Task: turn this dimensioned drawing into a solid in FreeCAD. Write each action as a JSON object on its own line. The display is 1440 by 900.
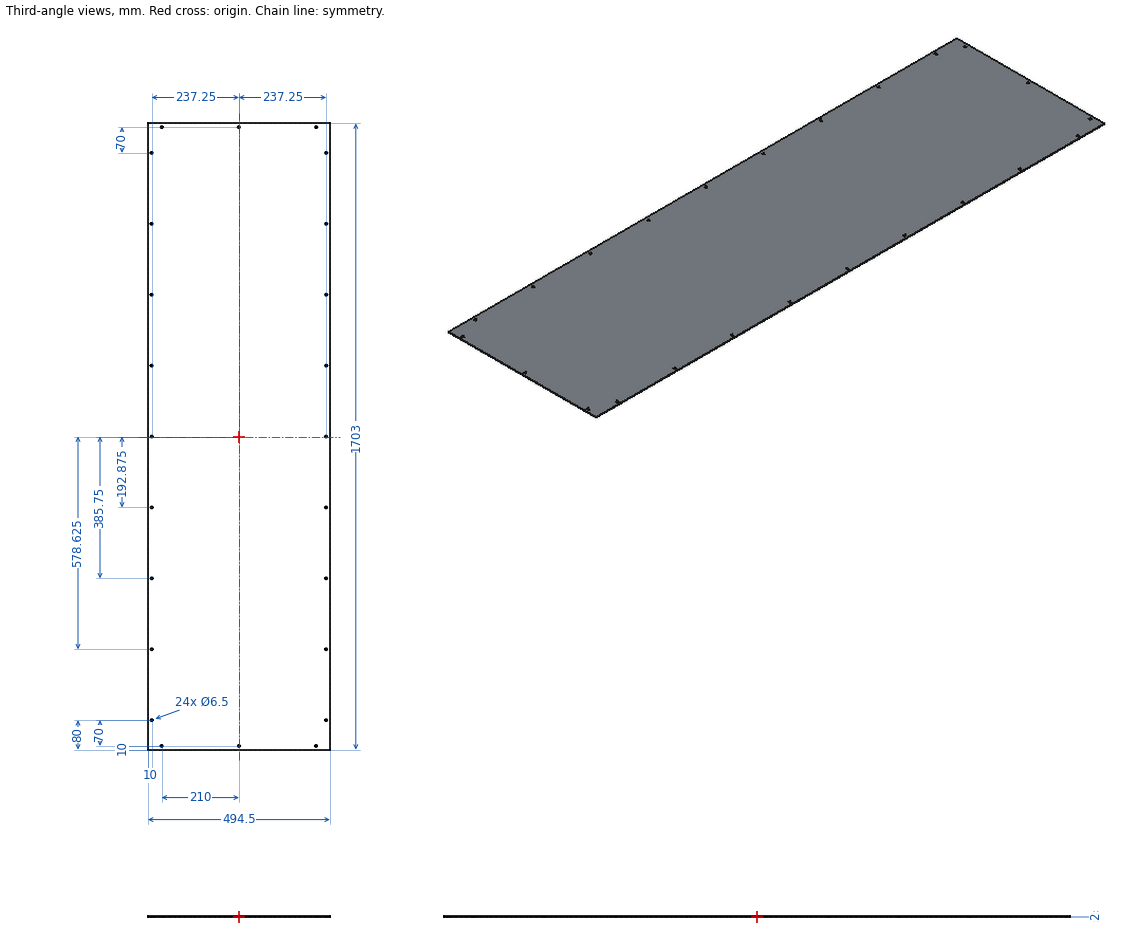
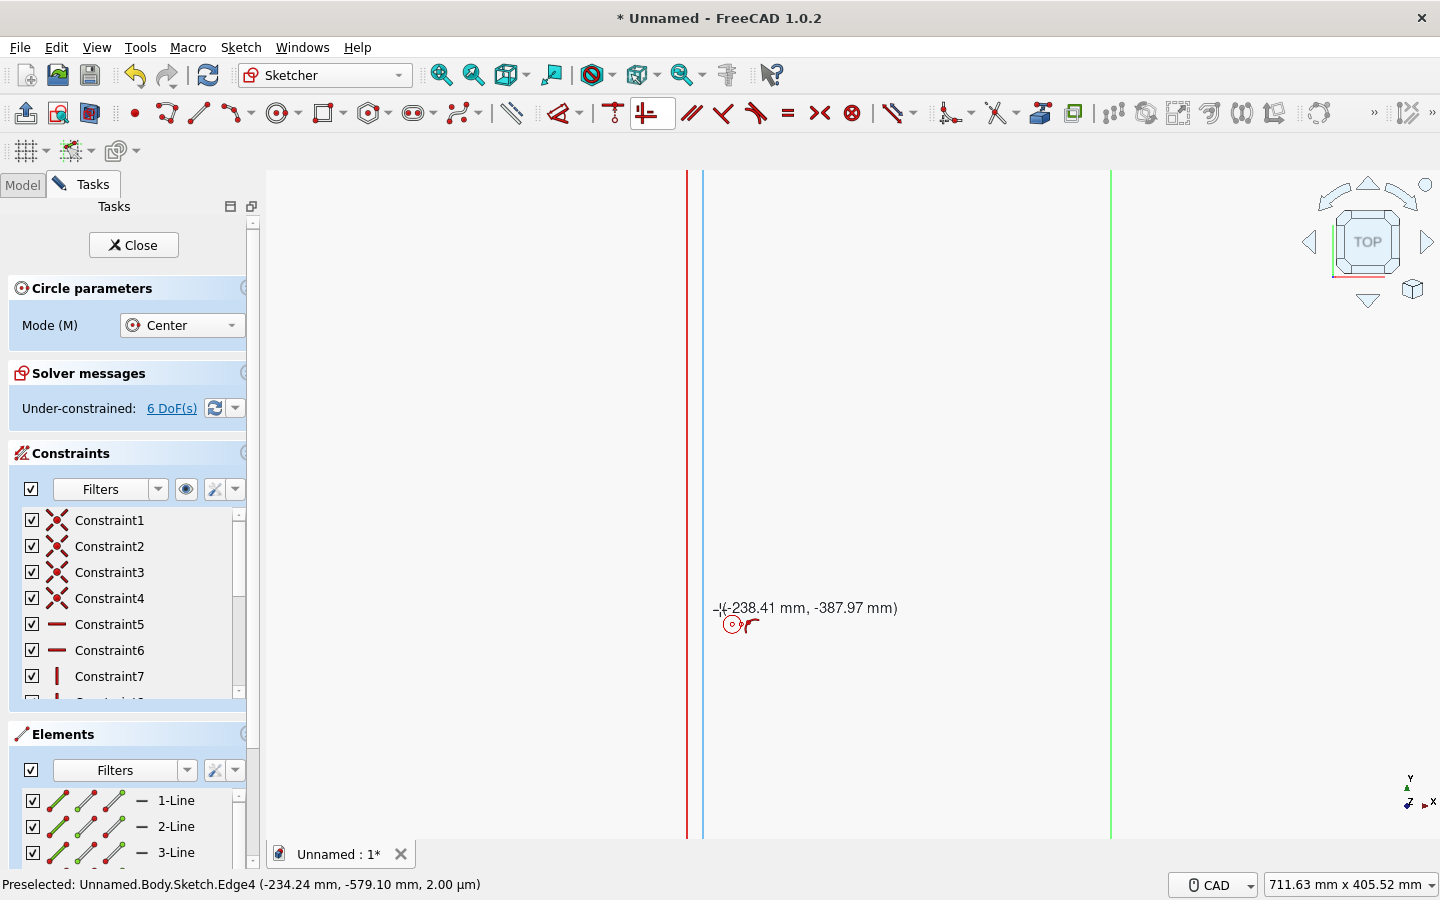
{"action": "left_click", "coordinate": [720, 609]}
{"action": "mouse_move", "coordinate": [724, 605]}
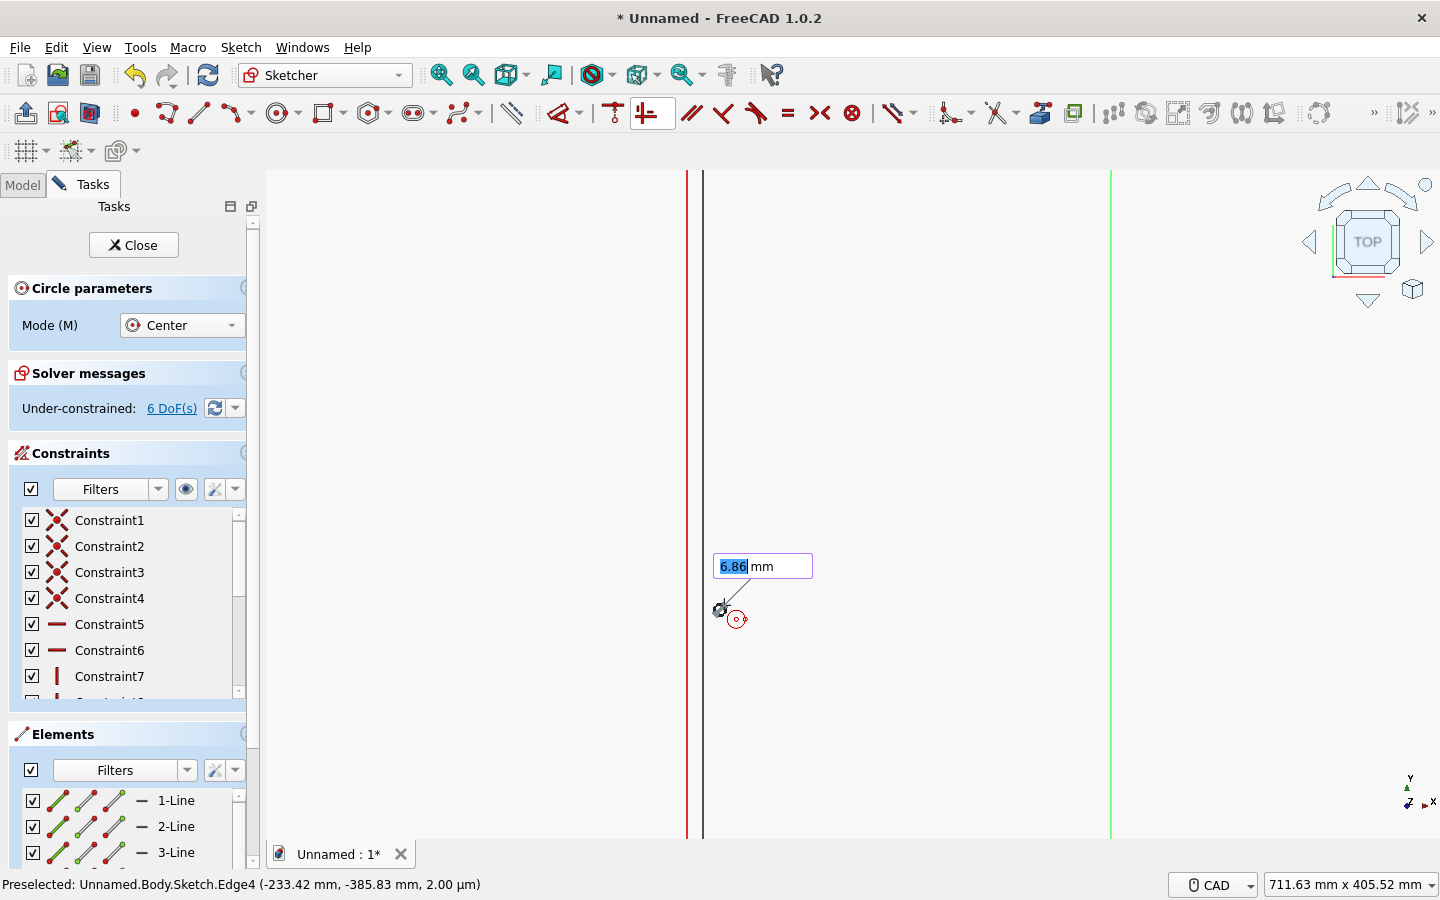
{"action": "type", "text": "6.5"}
{"action": "key", "text": "Return"}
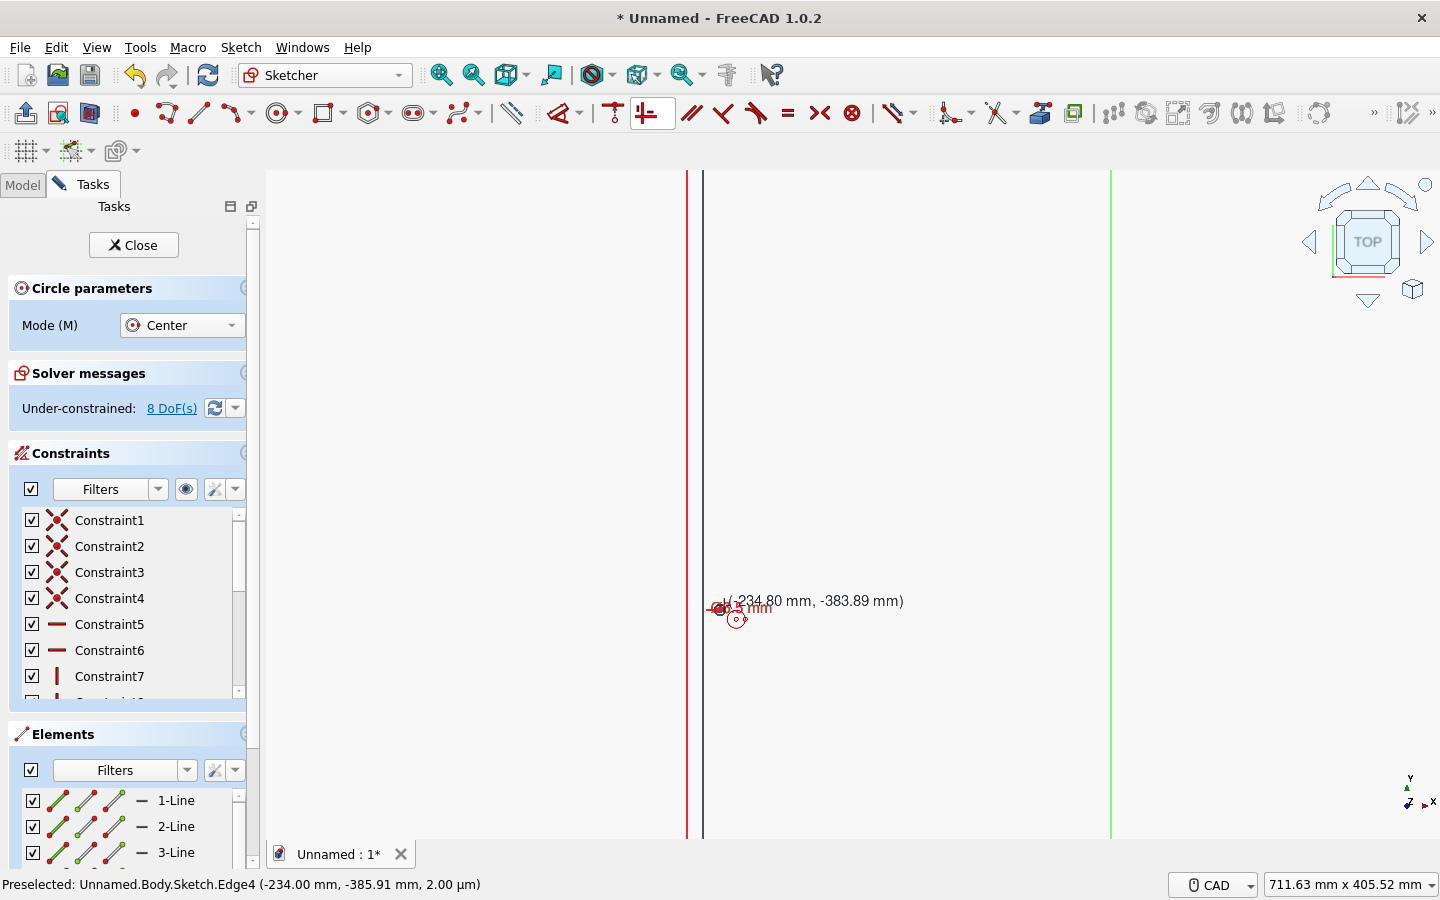
{"action": "scroll", "coordinate": [720, 291], "scroll_direction": "up", "scroll_amount": 8}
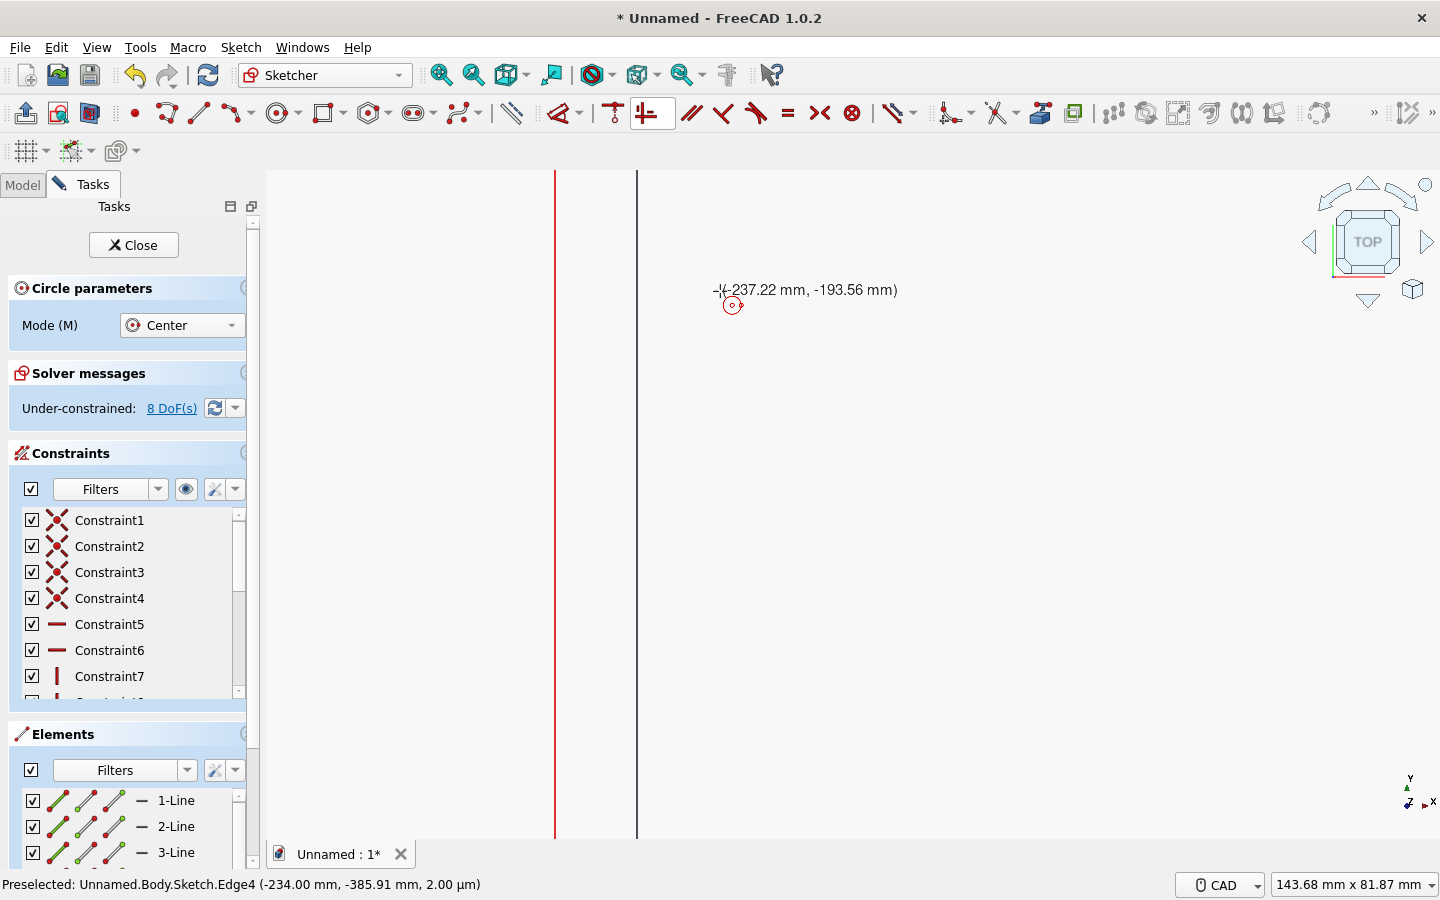
{"action": "scroll", "coordinate": [720, 566], "scroll_direction": "down", "scroll_amount": 17}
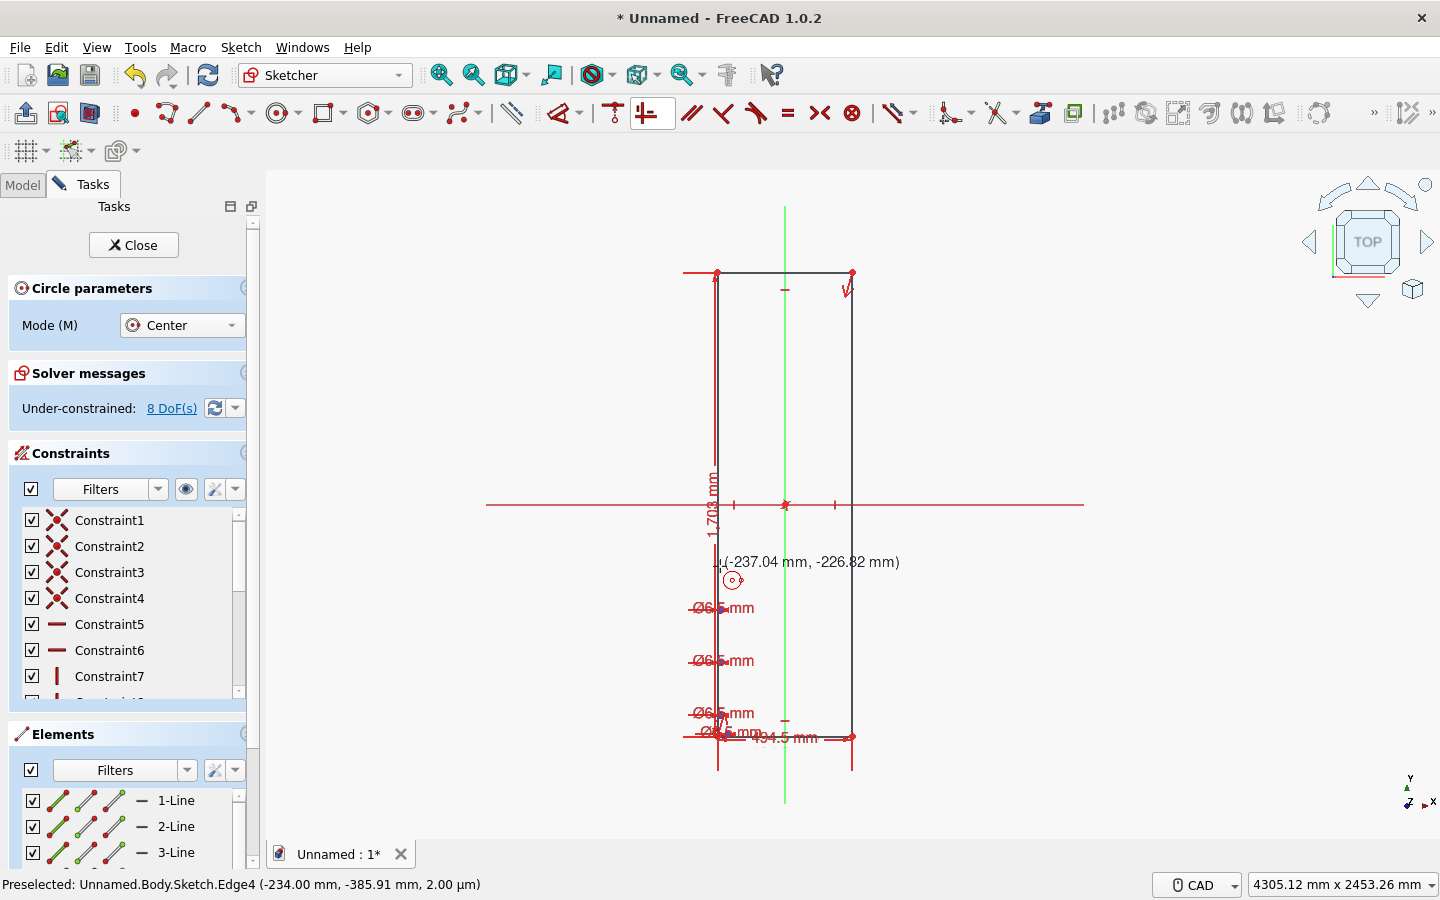
{"action": "scroll", "coordinate": [720, 557], "scroll_direction": "up", "scroll_amount": 9}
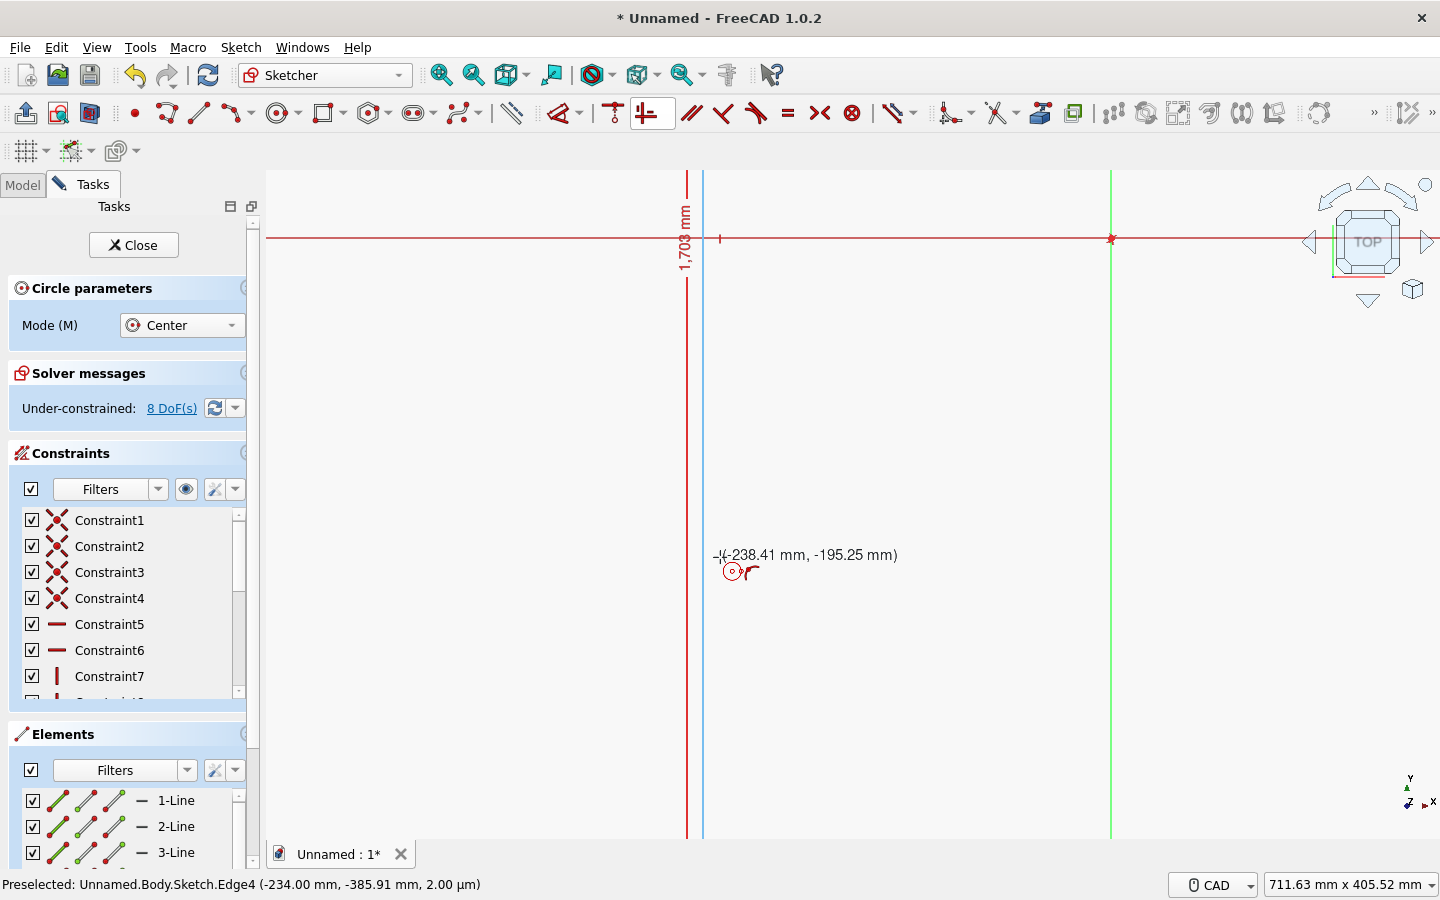
{"action": "left_click", "coordinate": [720, 556]}
{"action": "mouse_move", "coordinate": [724, 552]}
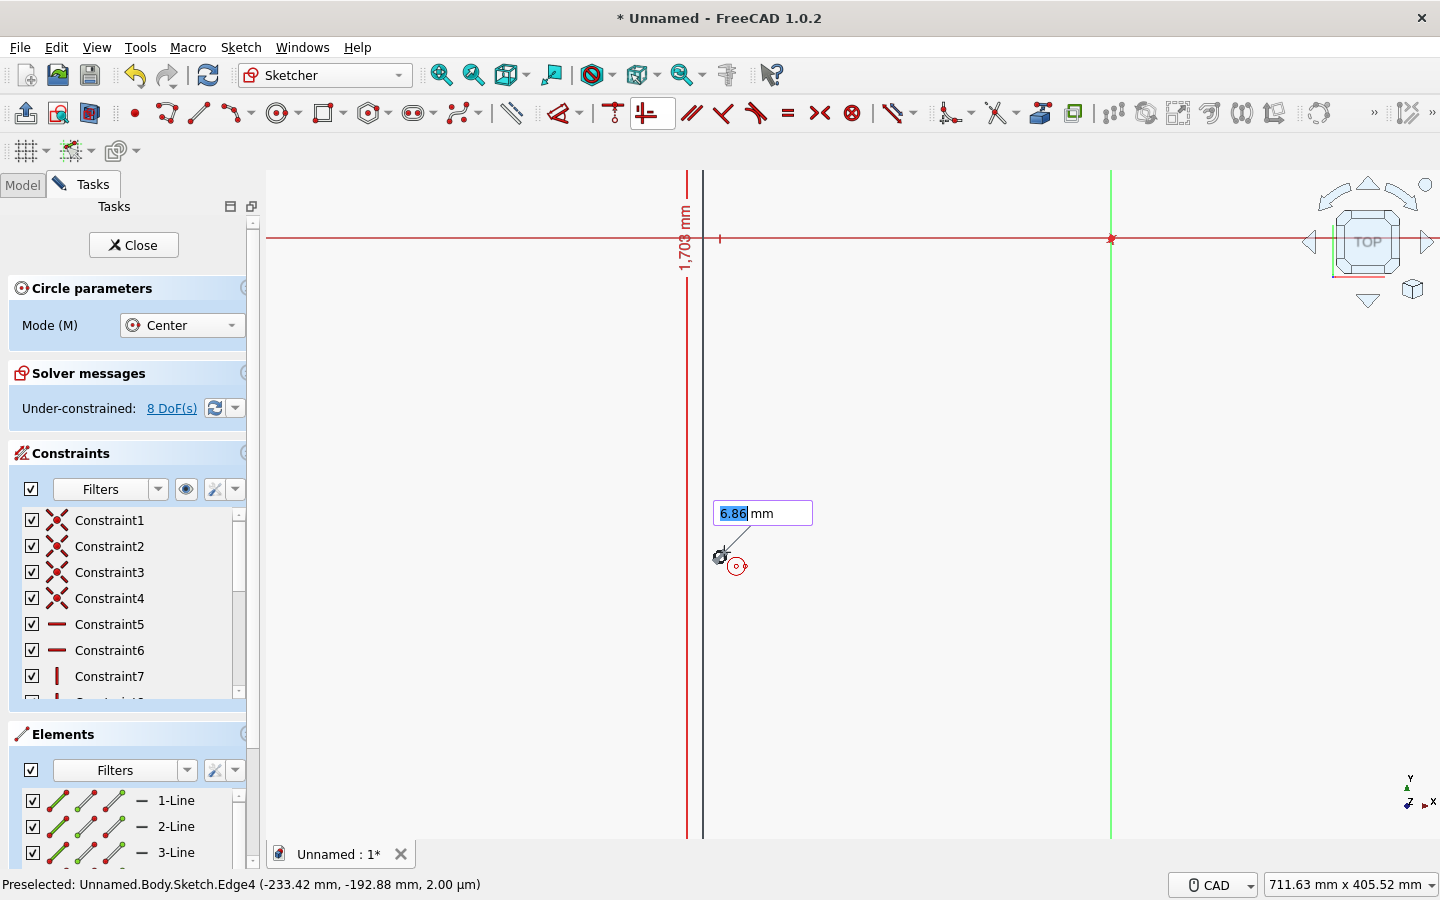
{"action": "type", "text": "6.5"}
{"action": "key", "text": "Return"}